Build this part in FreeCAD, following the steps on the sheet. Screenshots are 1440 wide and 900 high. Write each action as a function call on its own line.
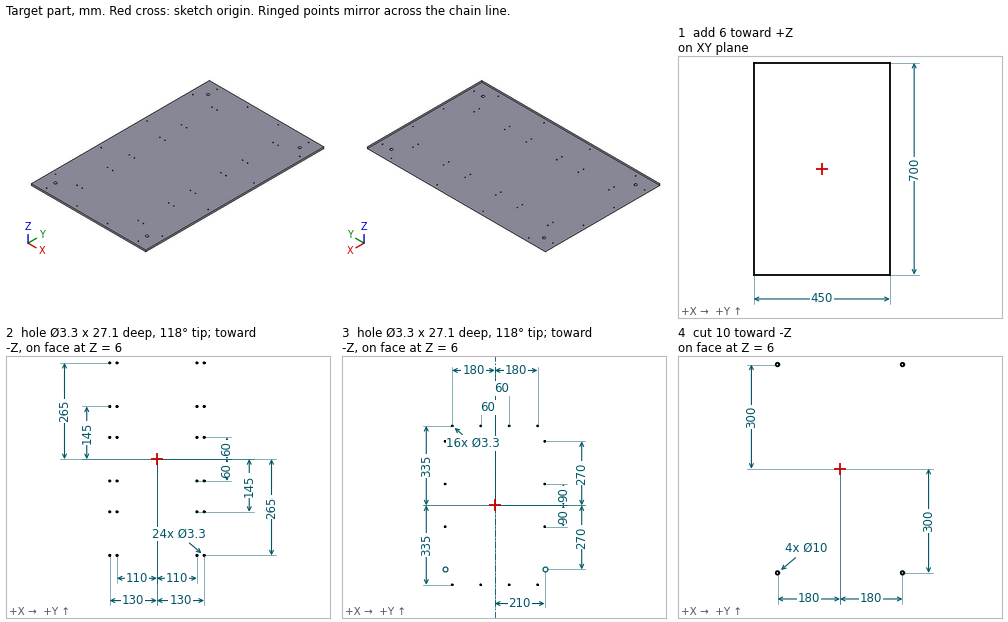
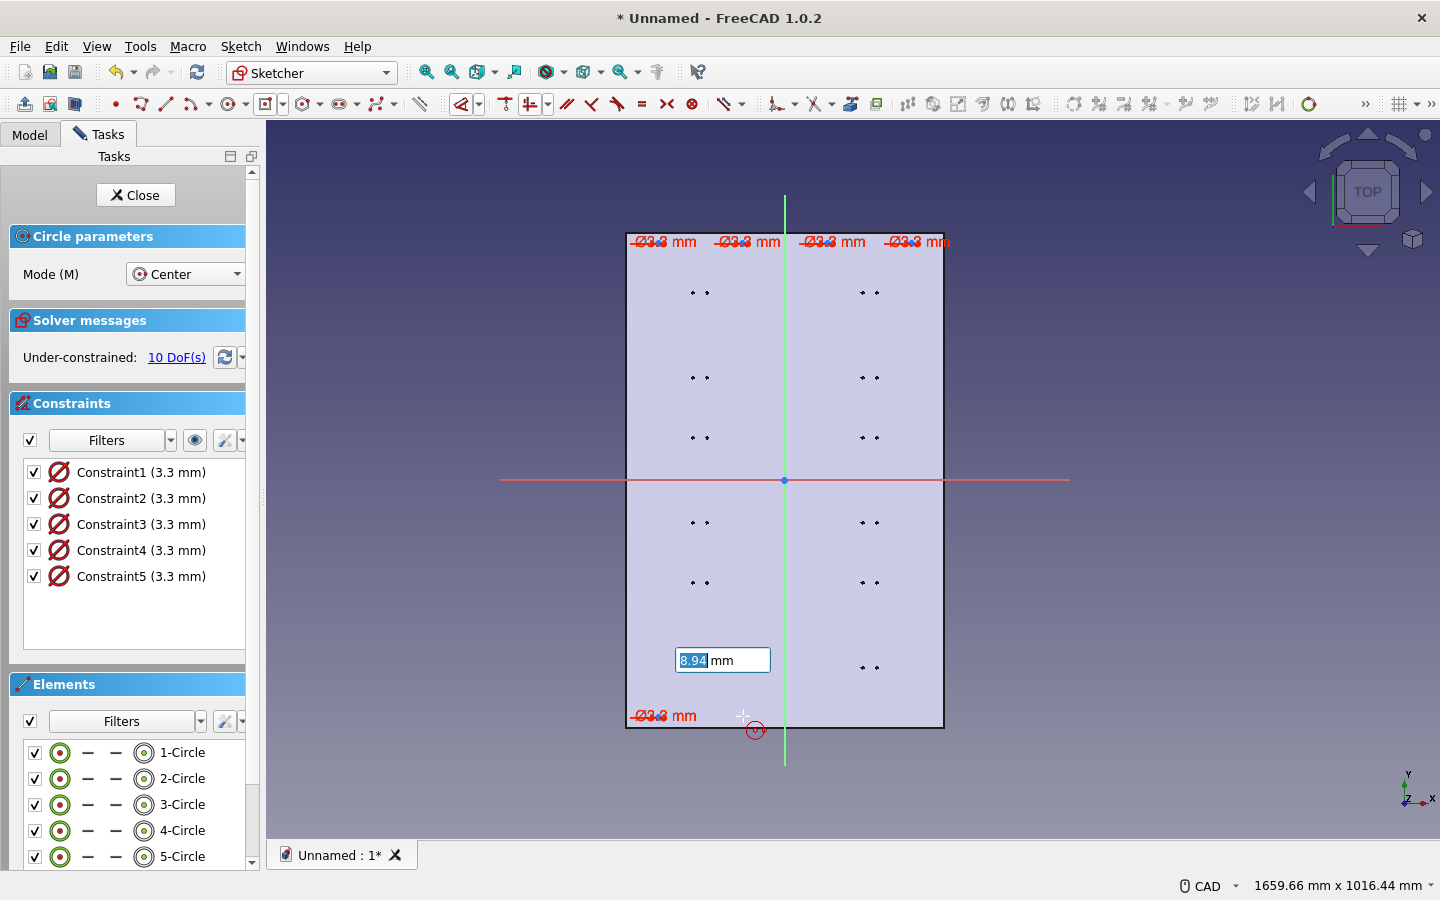
text(3.3)
key(Return)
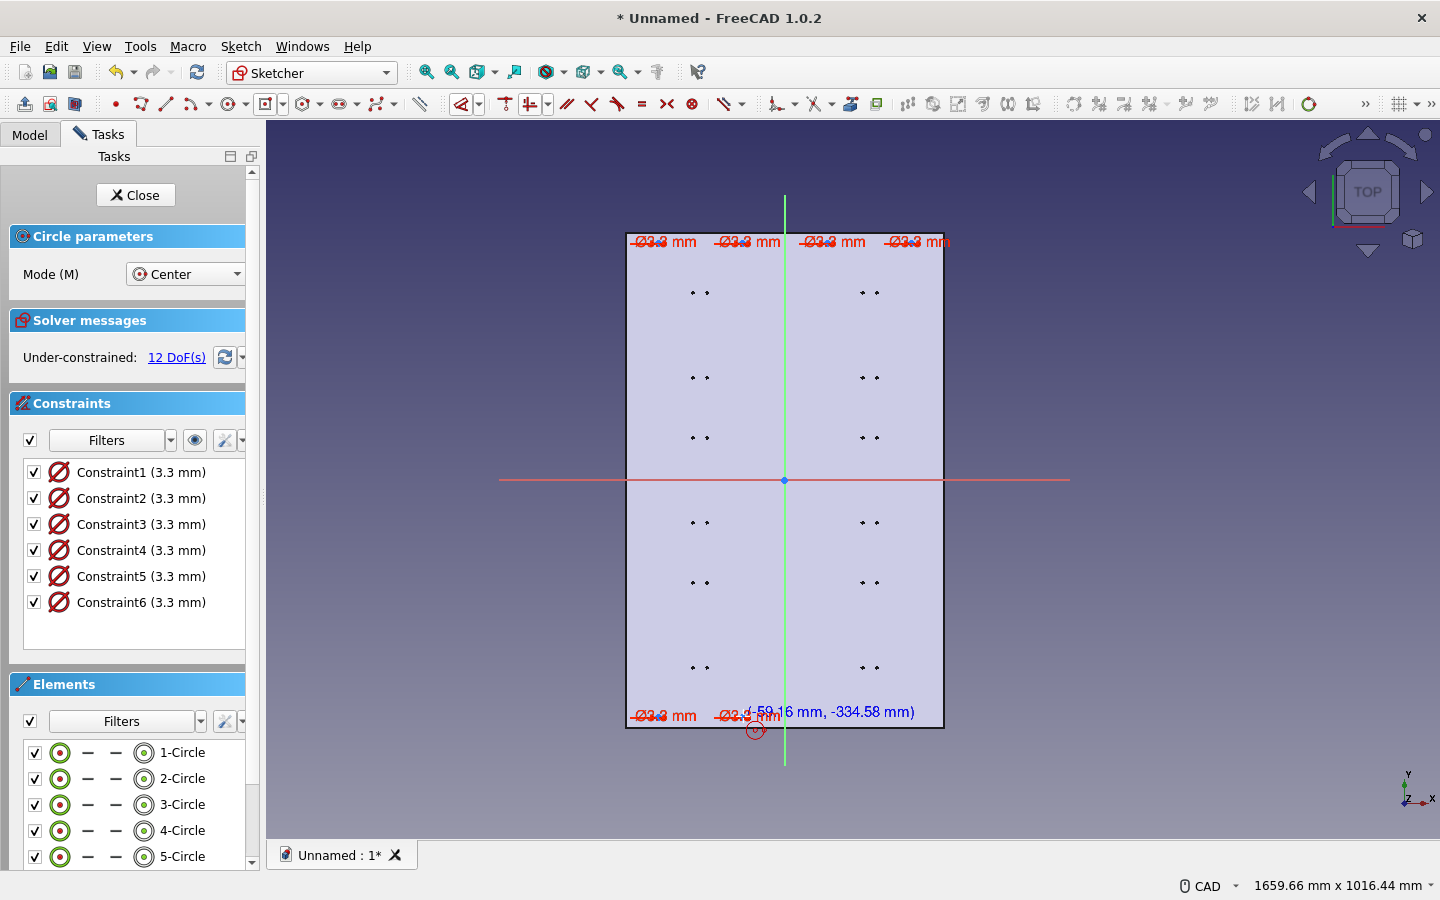
scroll(827, 717, up, 15)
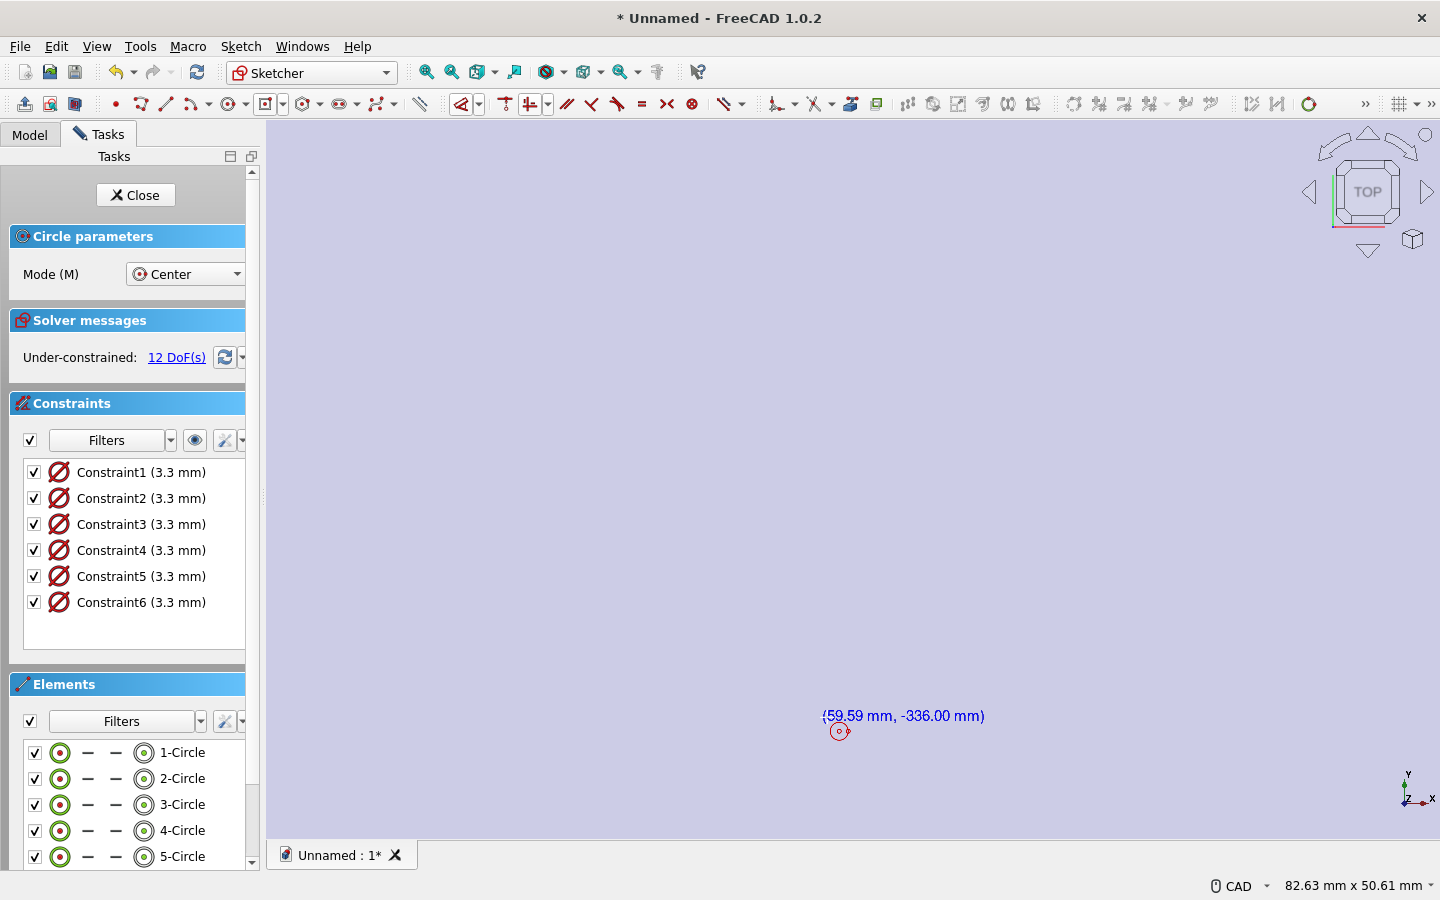
scroll(827, 717, down, 15)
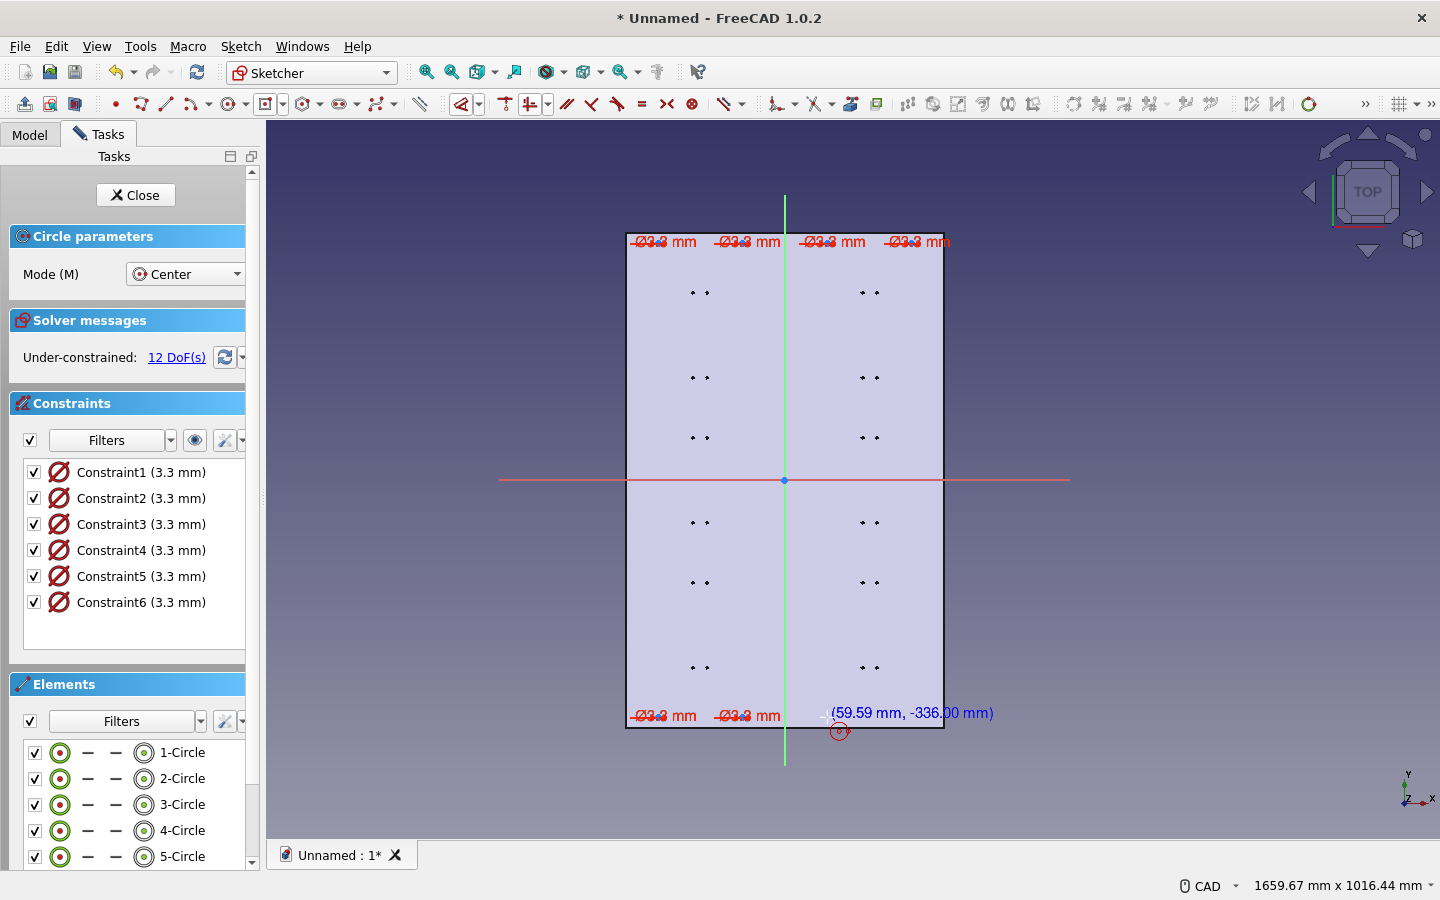
click(827, 717)
move(828, 716)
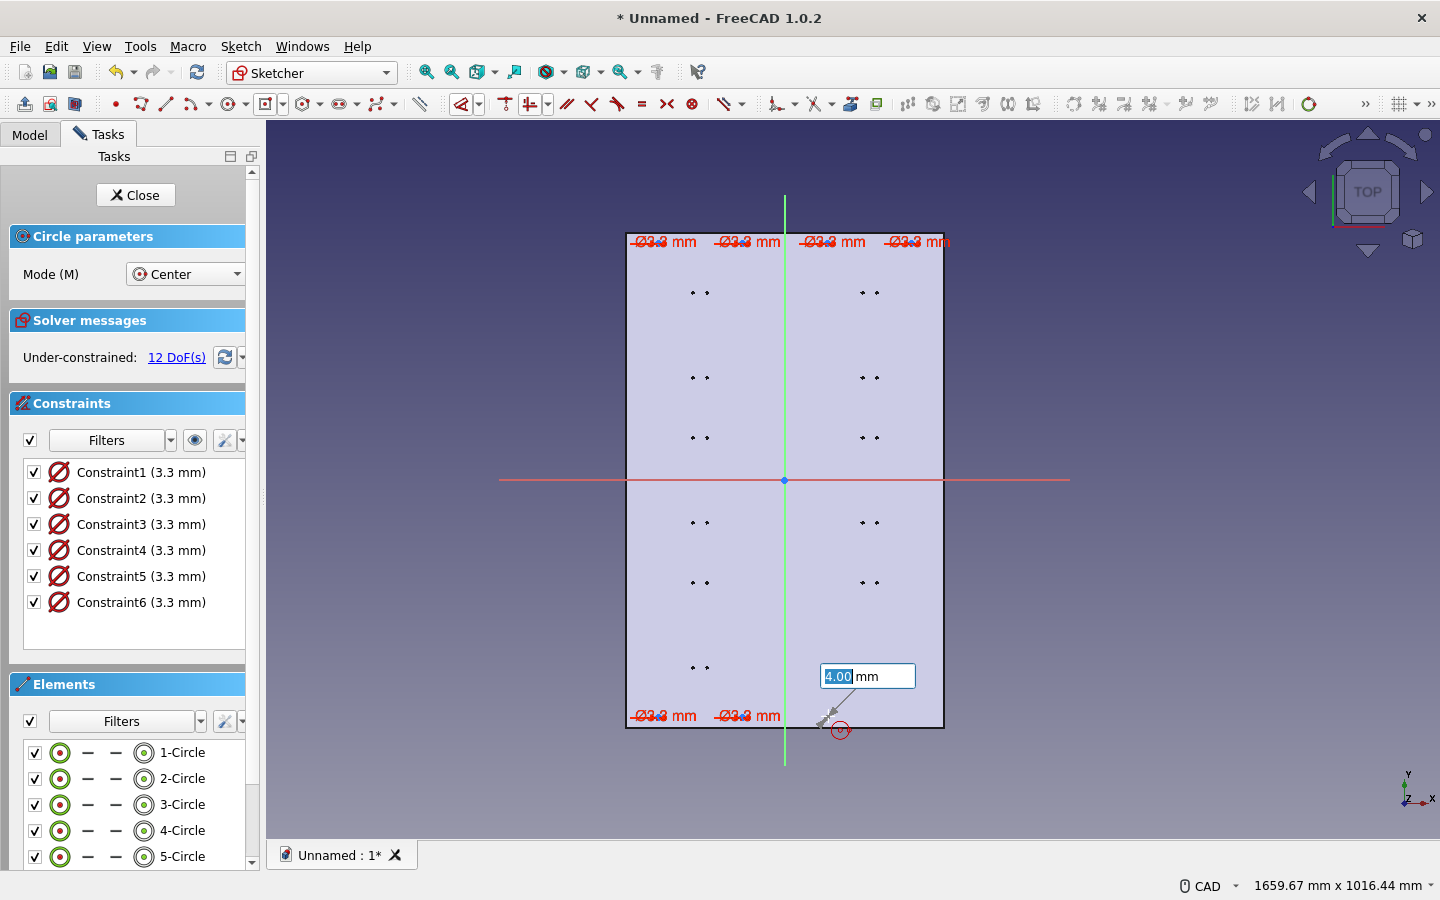
text(3.3)
key(Return)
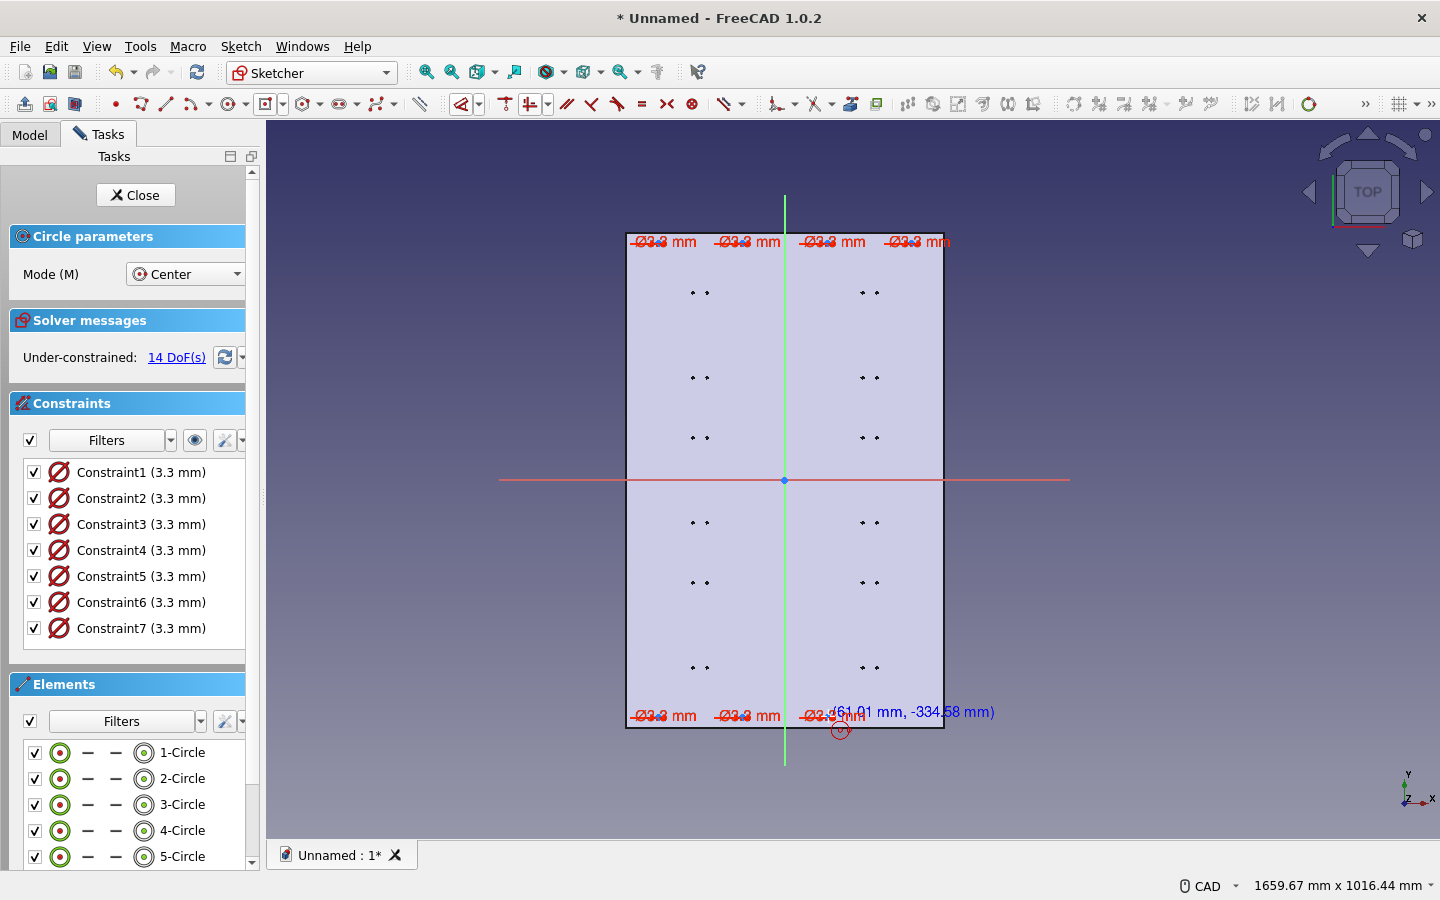
scroll(912, 717, up, 15)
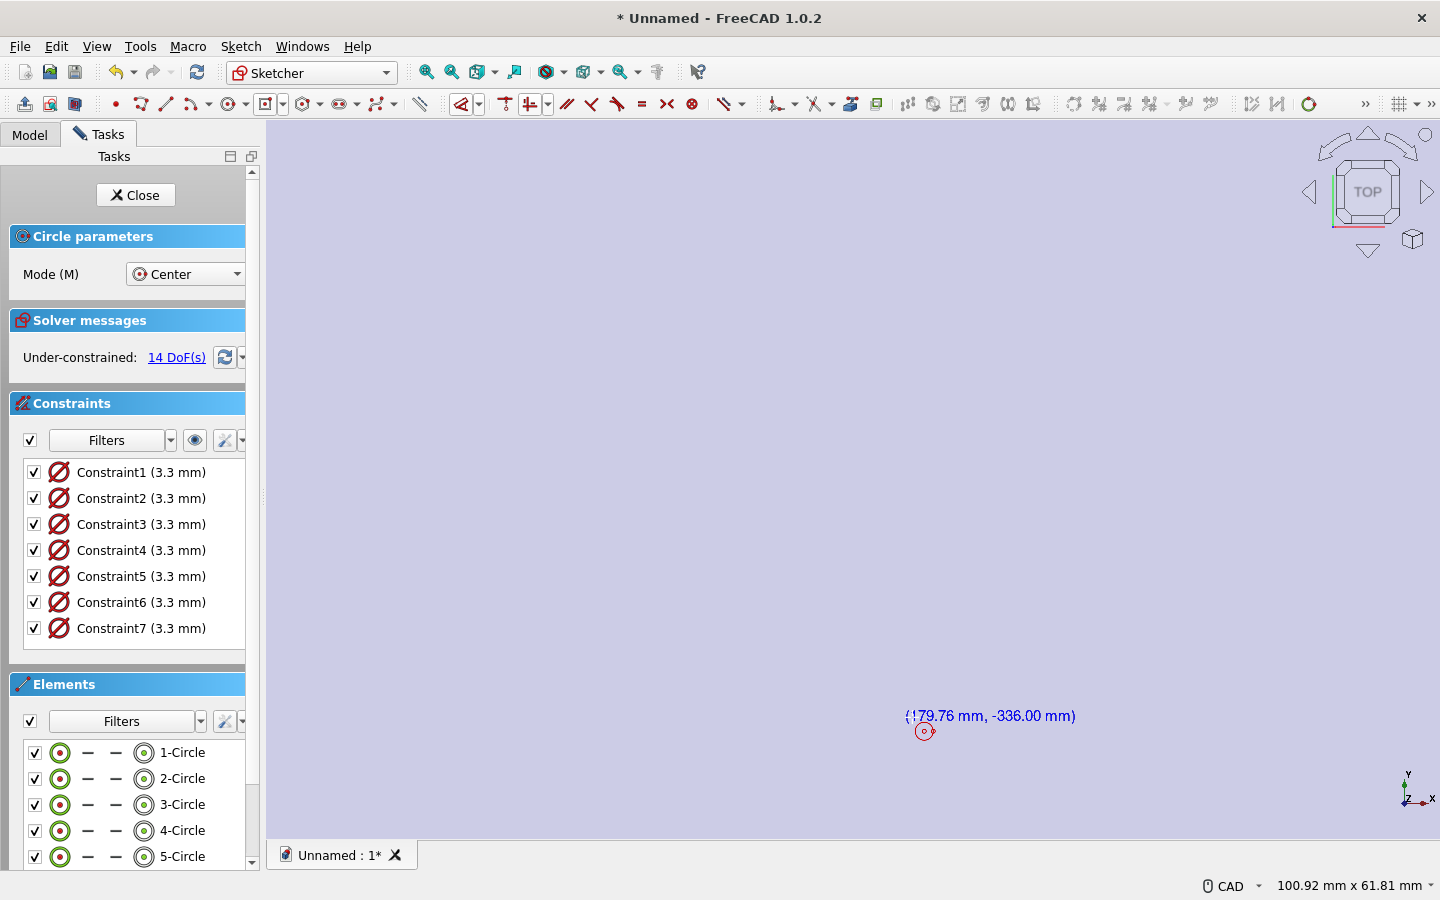
scroll(912, 717, down, 15)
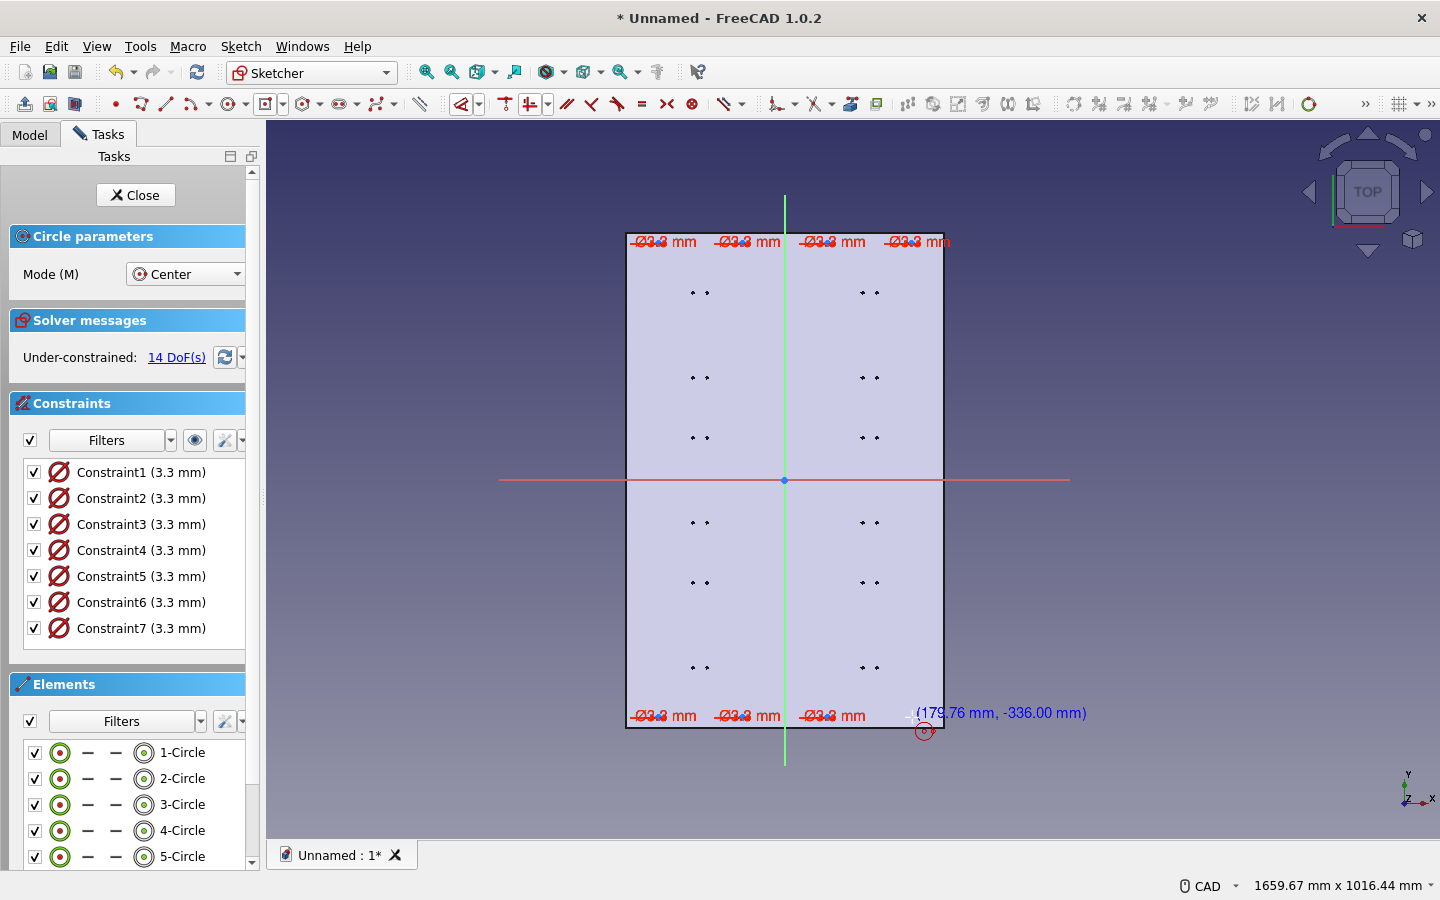
click(912, 717)
move(913, 716)